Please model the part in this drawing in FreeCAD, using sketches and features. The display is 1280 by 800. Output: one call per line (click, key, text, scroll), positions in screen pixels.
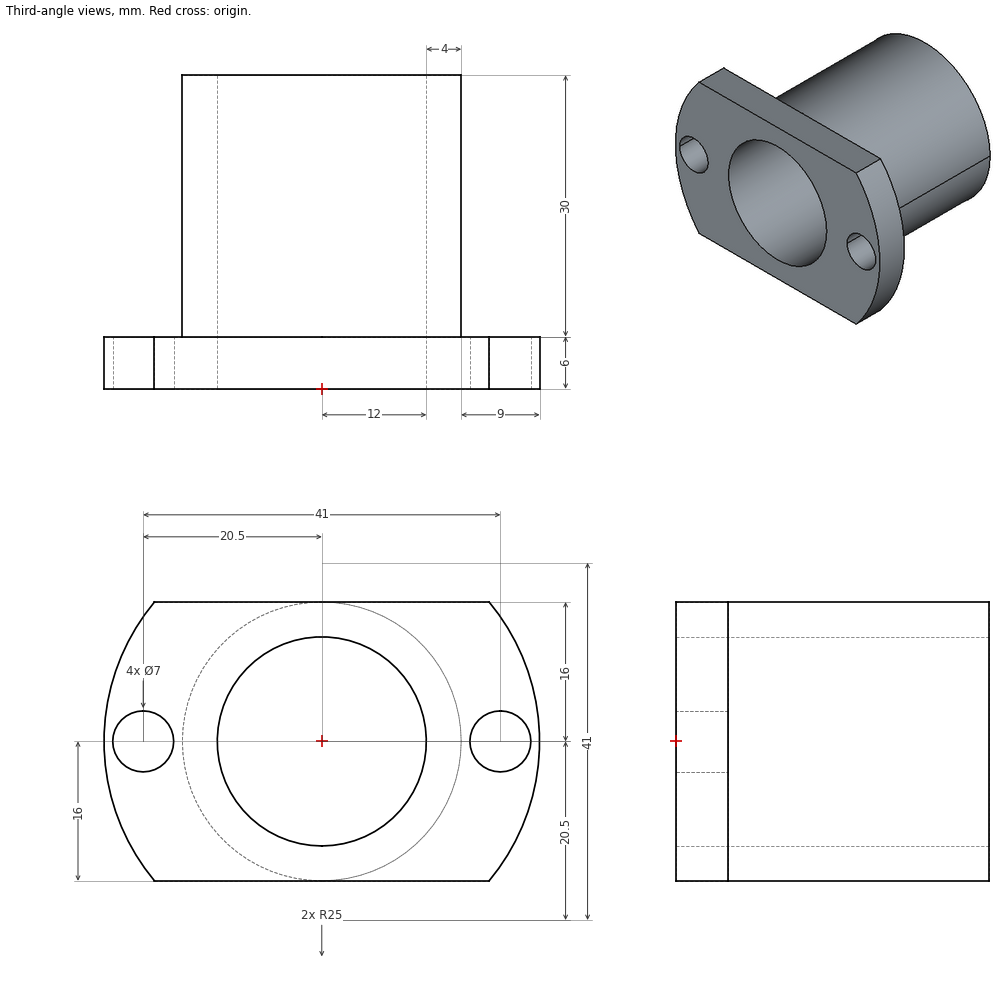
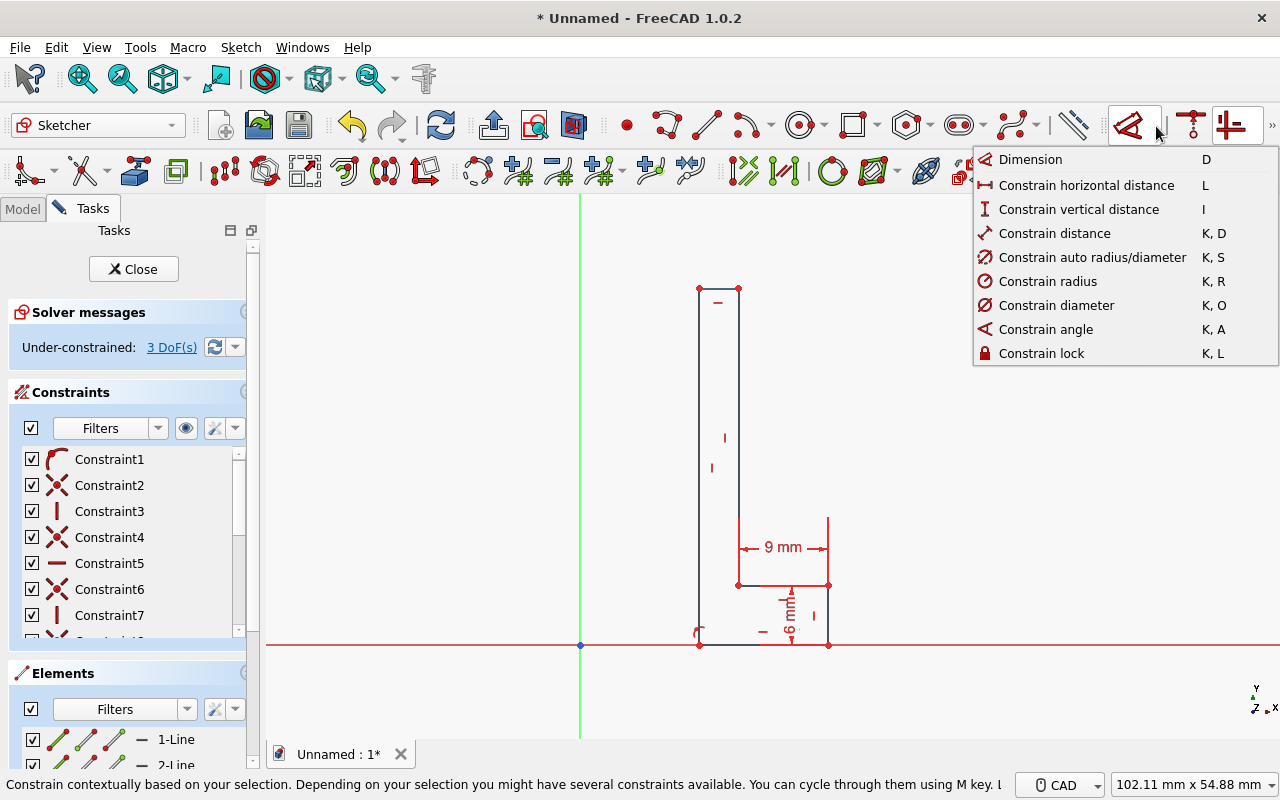
click(1126, 185)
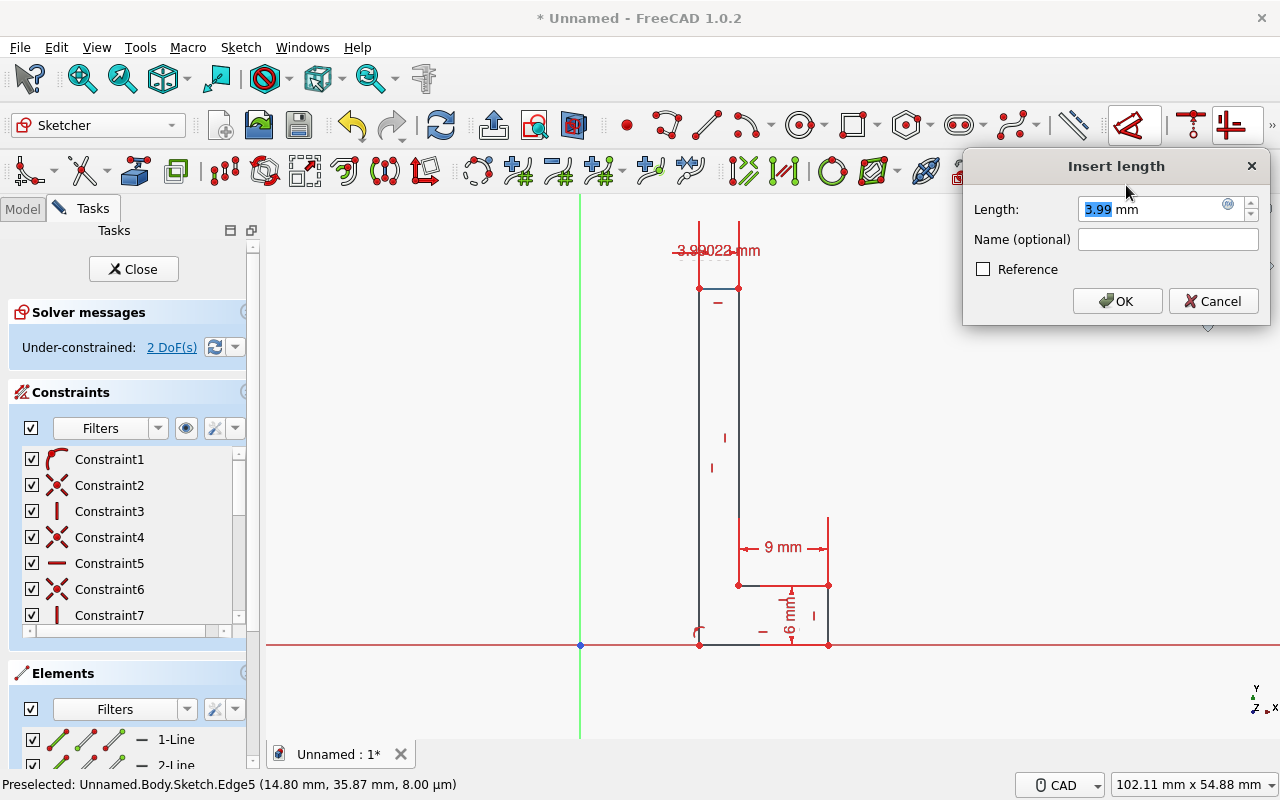
text(4)
key(Return)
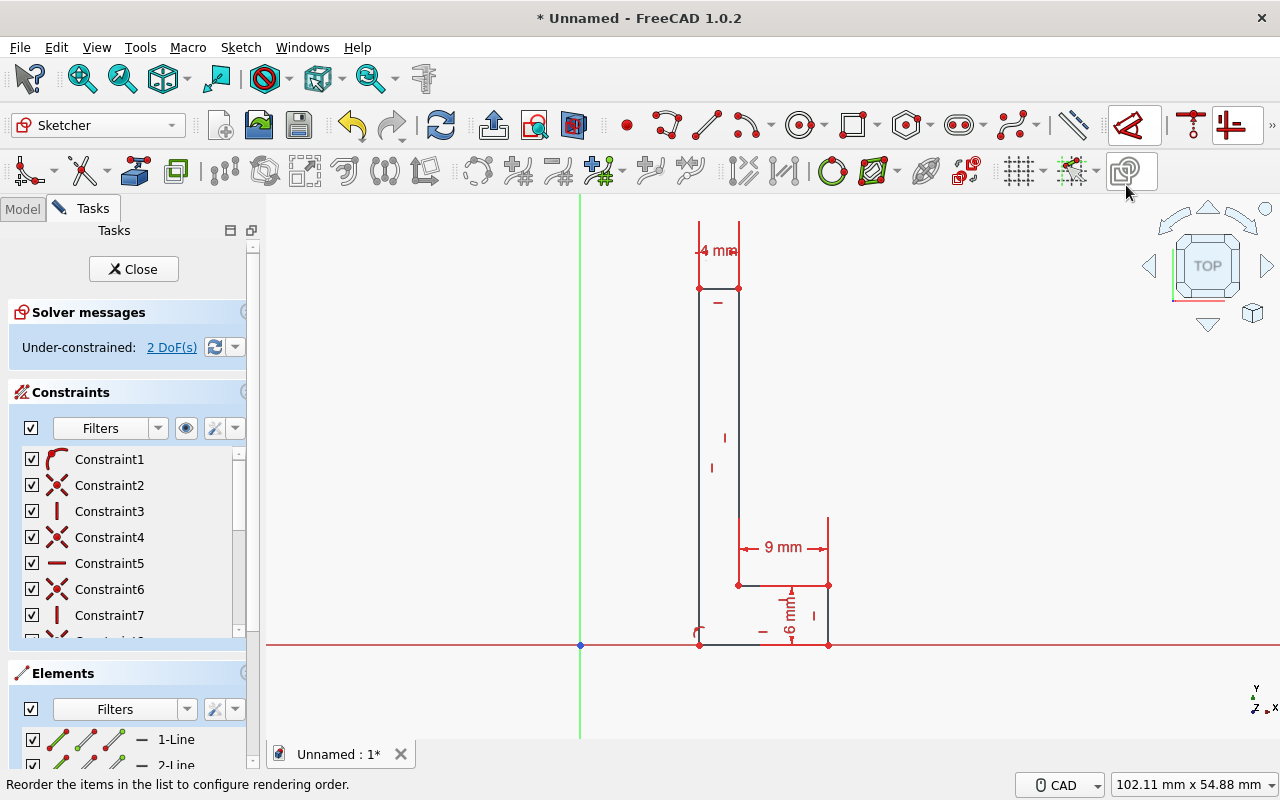
click(739, 497)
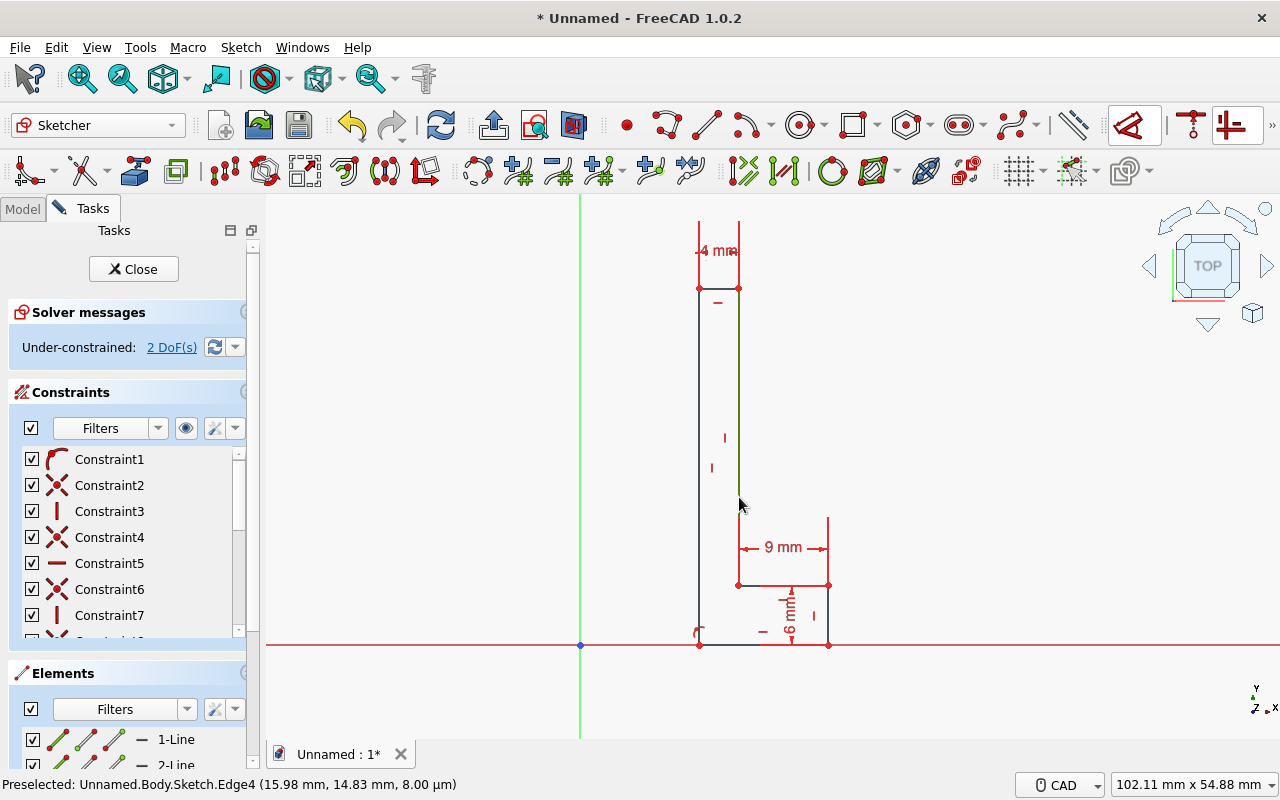
click(1156, 126)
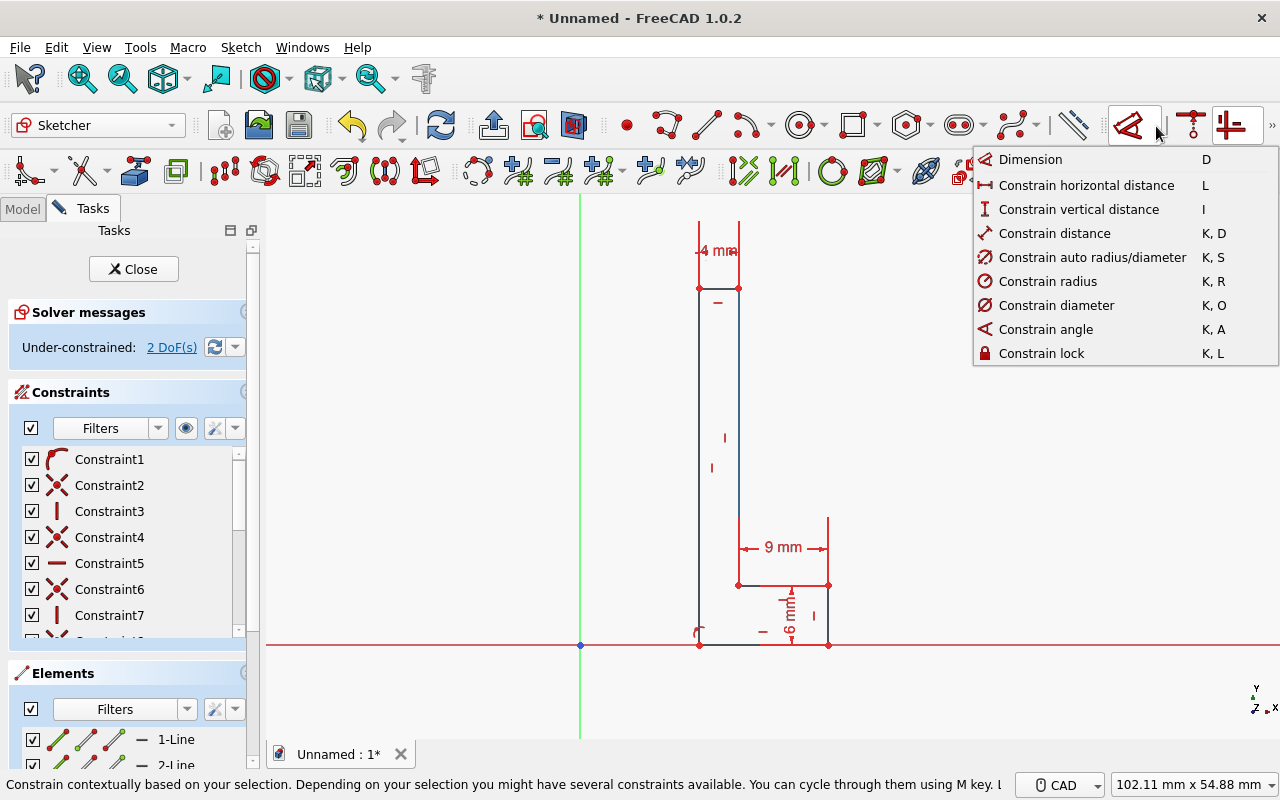
click(1126, 209)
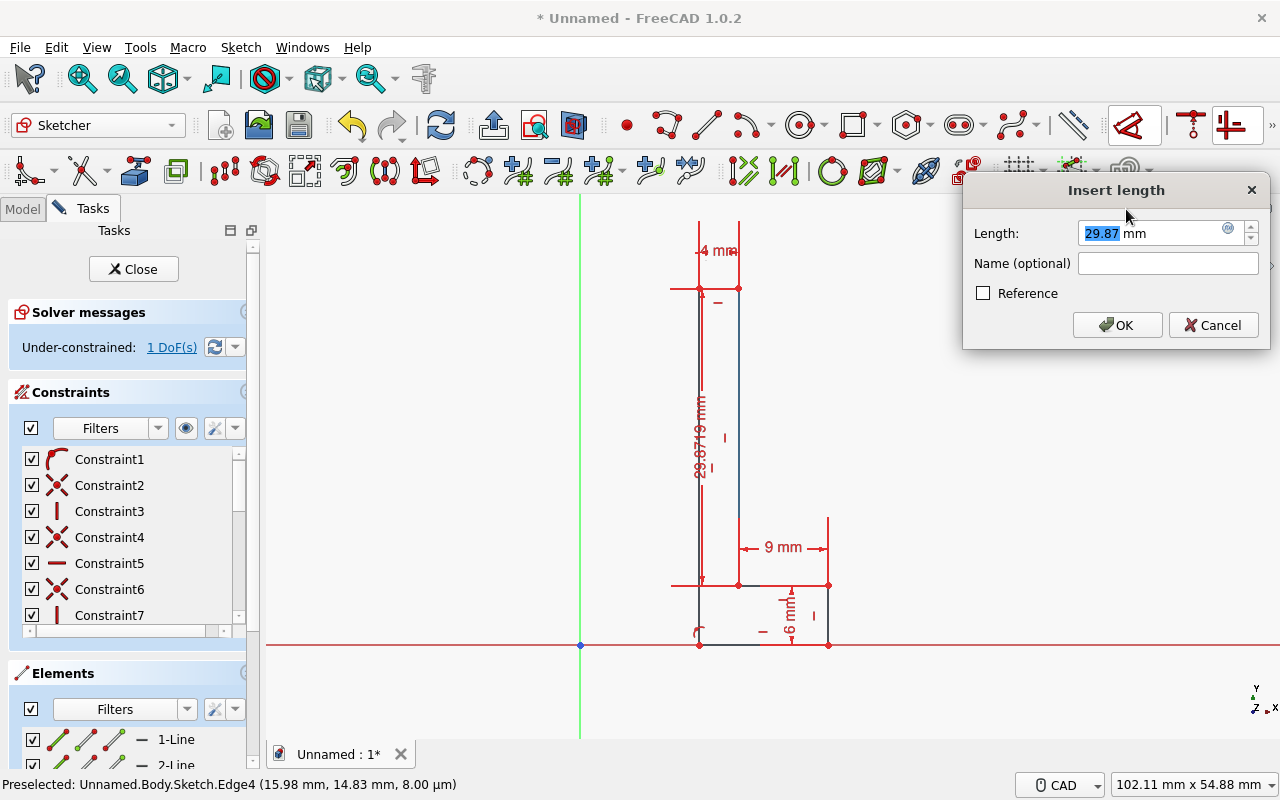
text(30)
key(Return)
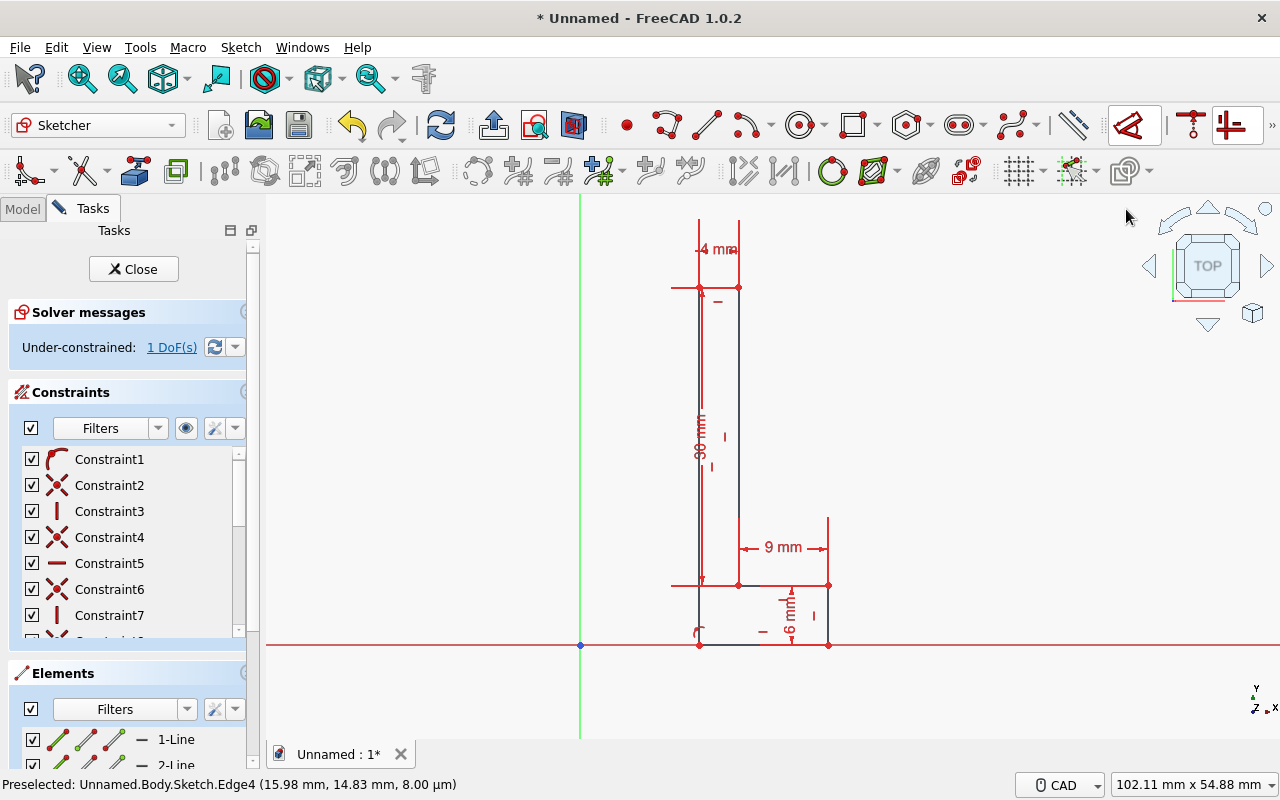
click(699, 645)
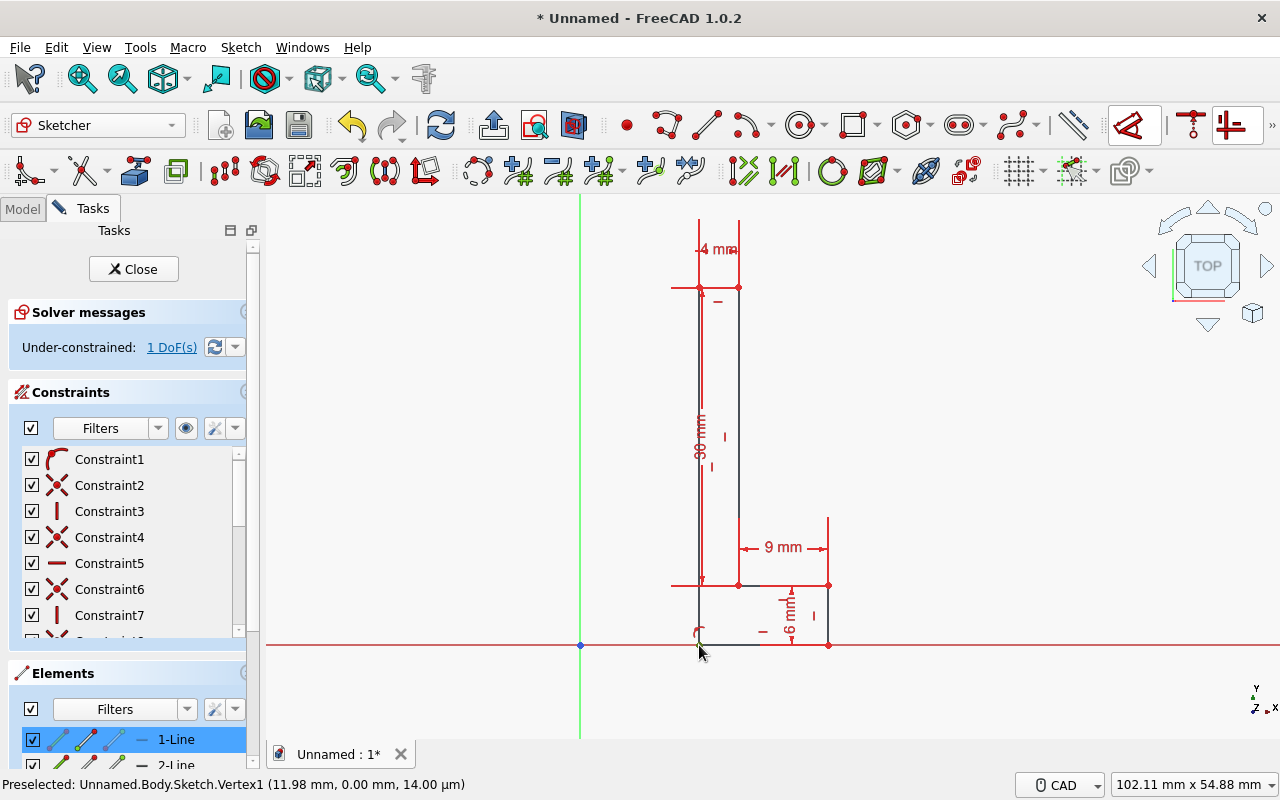
key(l)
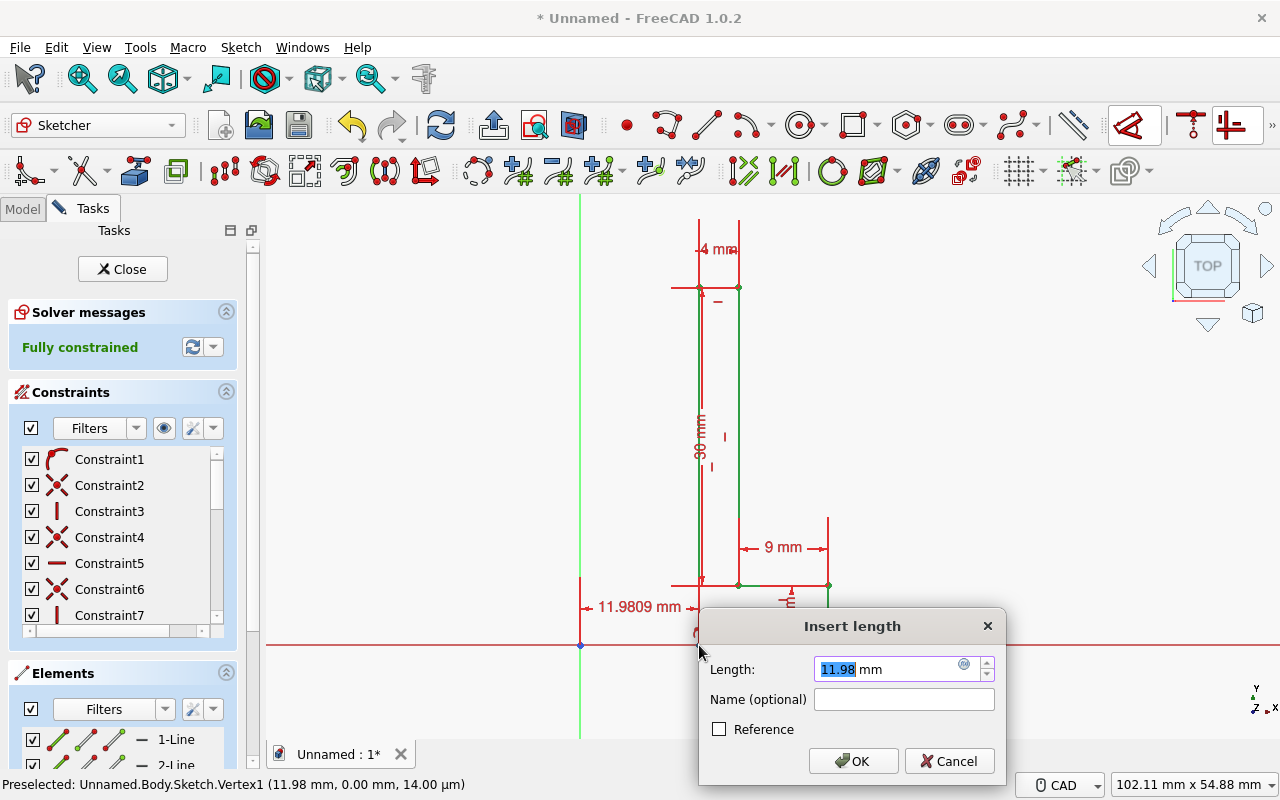
text(12)
key(Return)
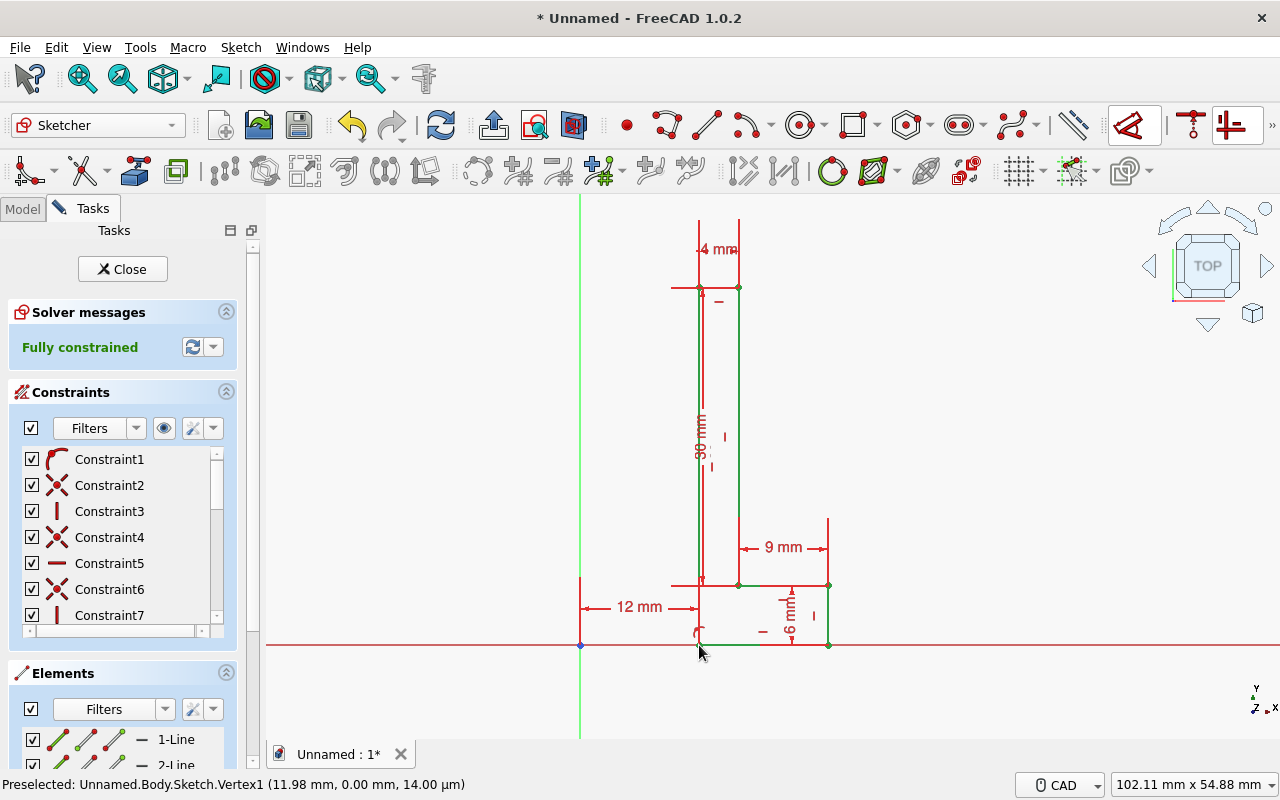
click(123, 269)